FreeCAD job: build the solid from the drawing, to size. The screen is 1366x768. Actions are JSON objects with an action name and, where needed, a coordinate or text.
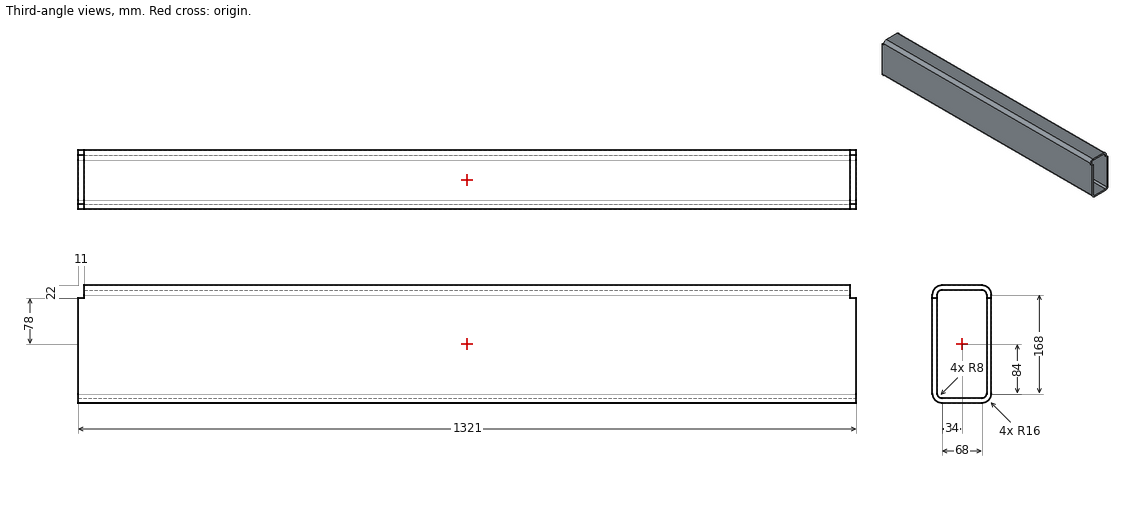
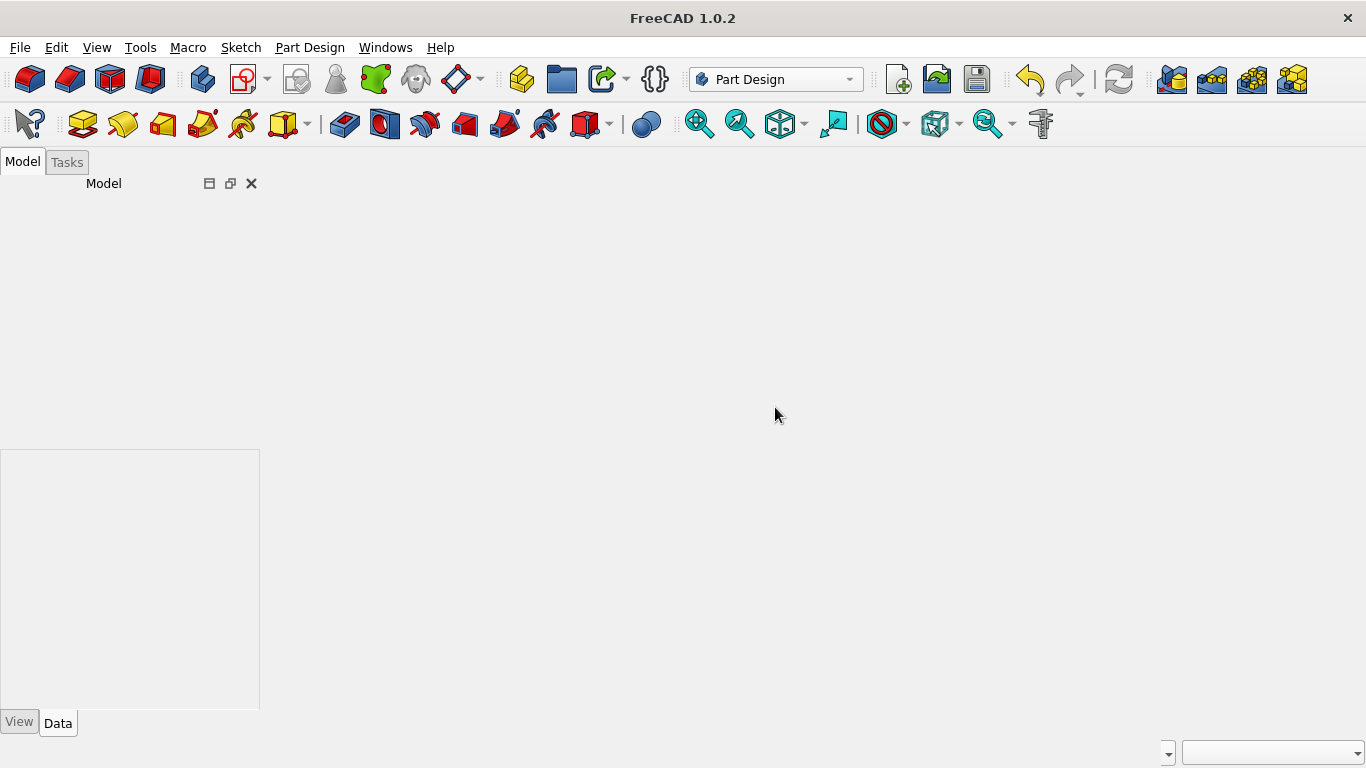
{"action": "left_click", "coordinate": [898, 80]}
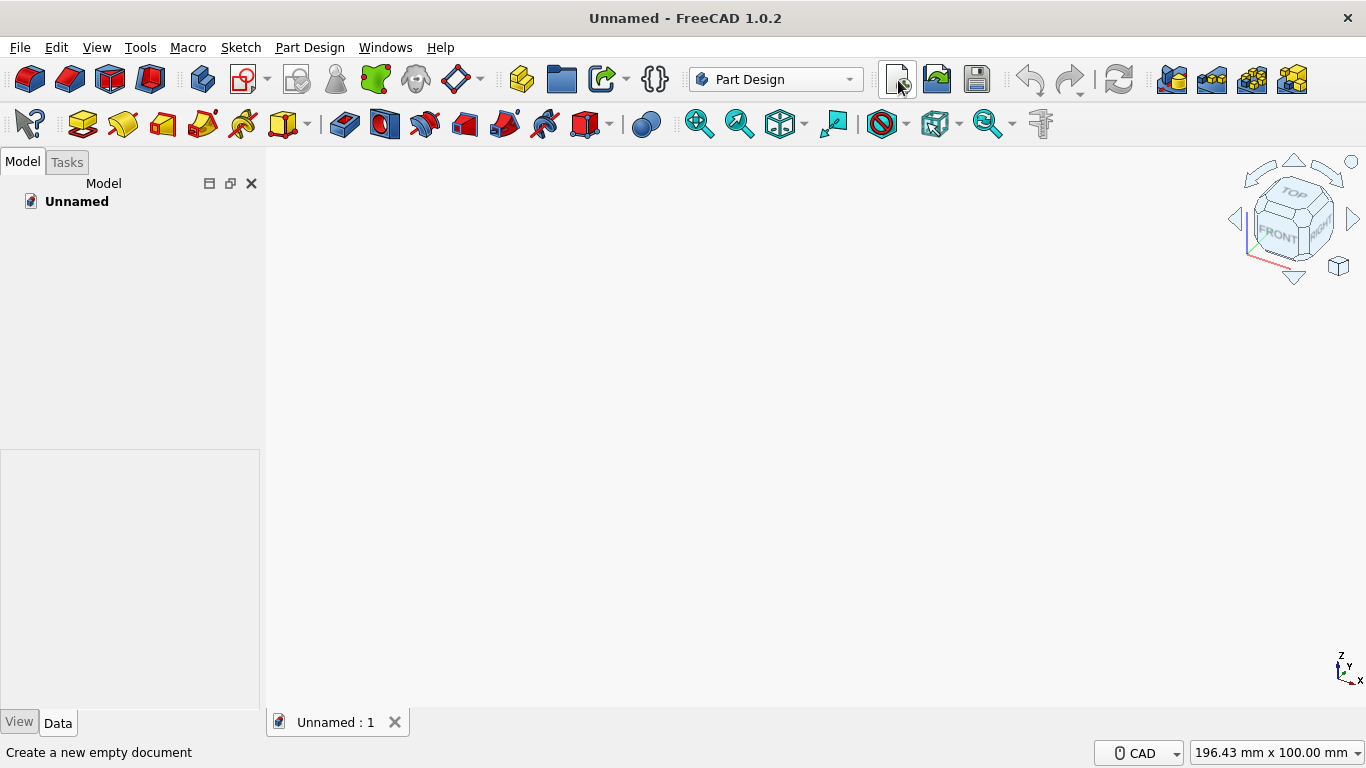
{"action": "left_click", "coordinate": [204, 80]}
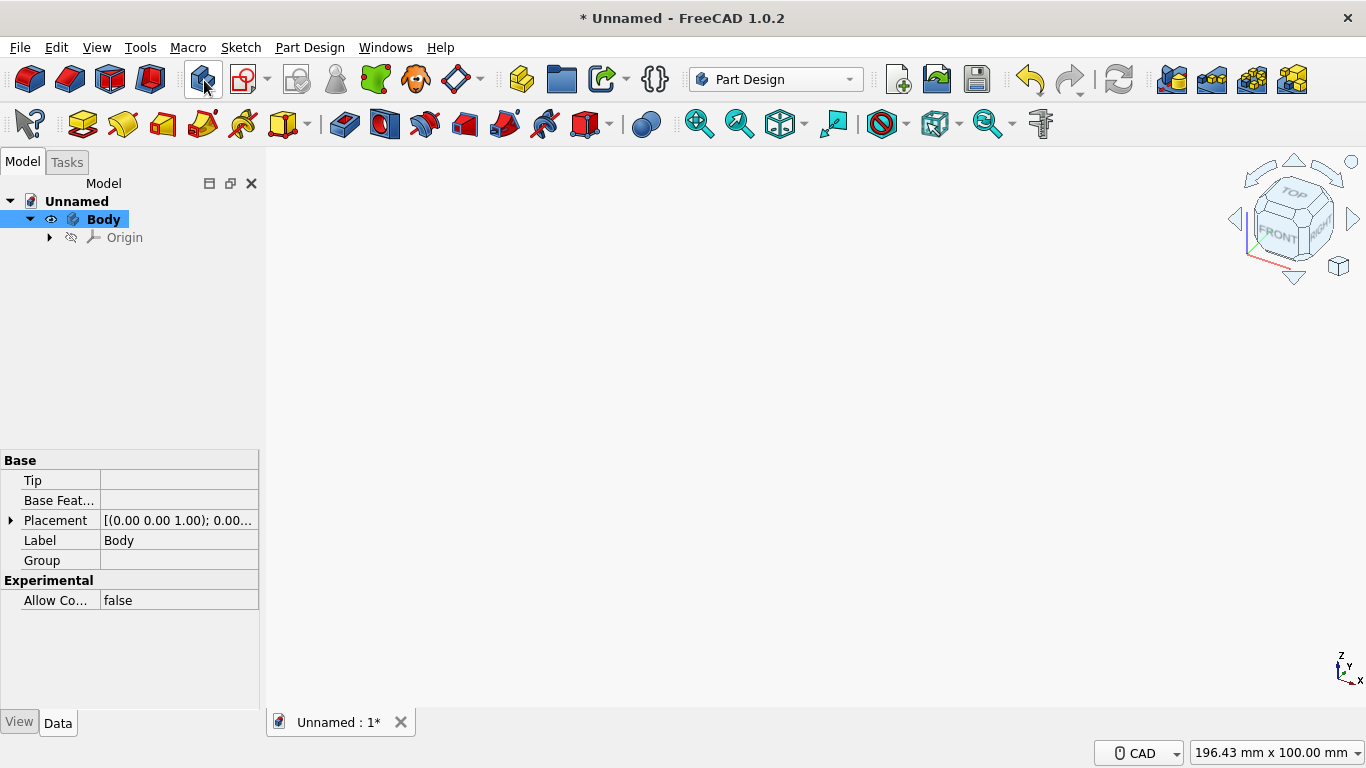
{"action": "left_click", "coordinate": [50, 237]}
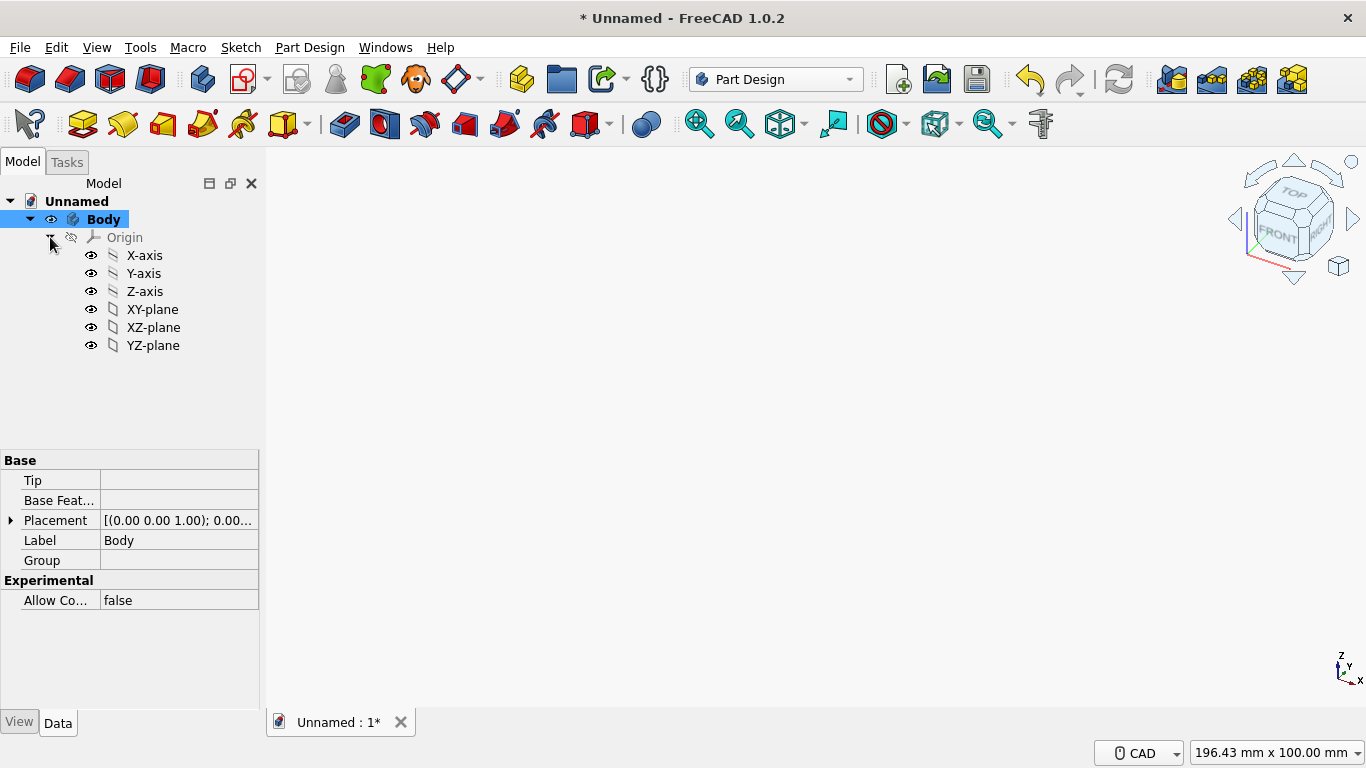
{"action": "left_click", "coordinate": [136, 345]}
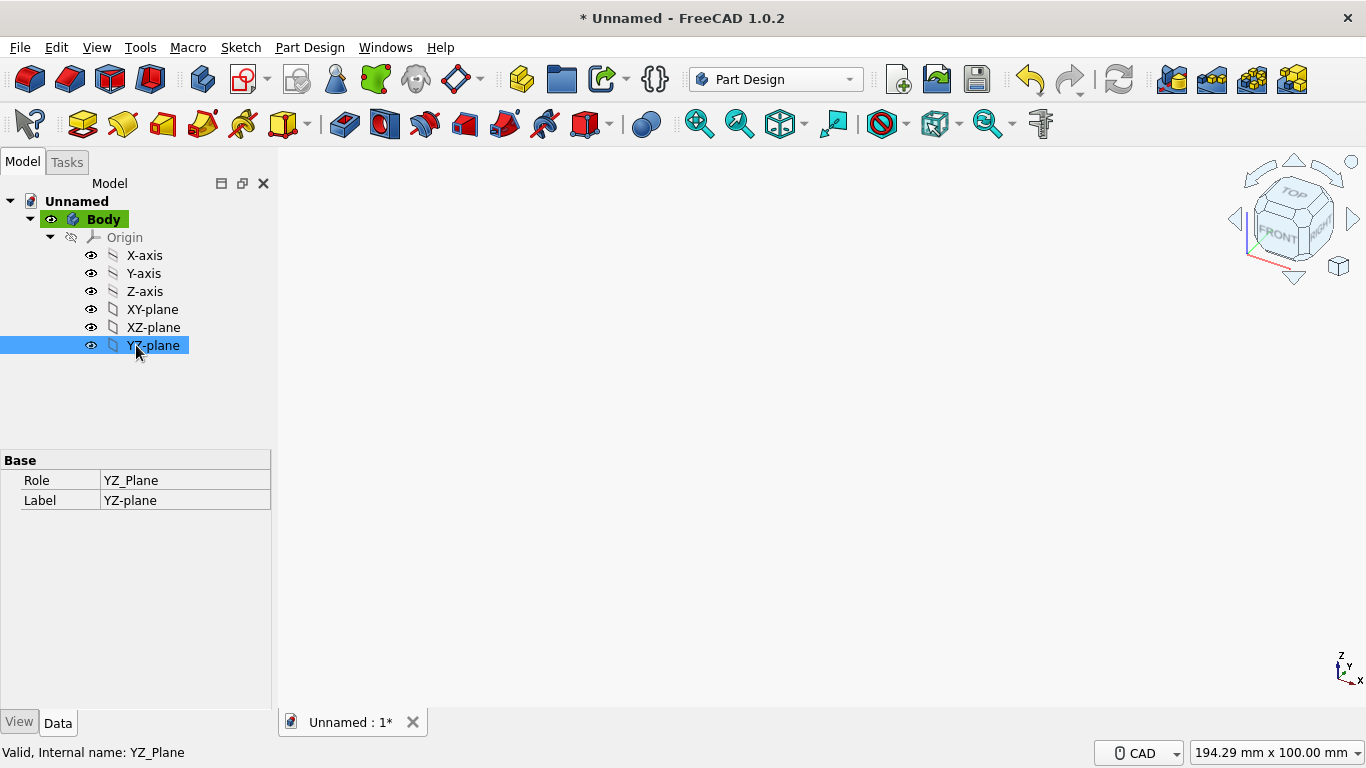
{"action": "left_click", "coordinate": [456, 80]}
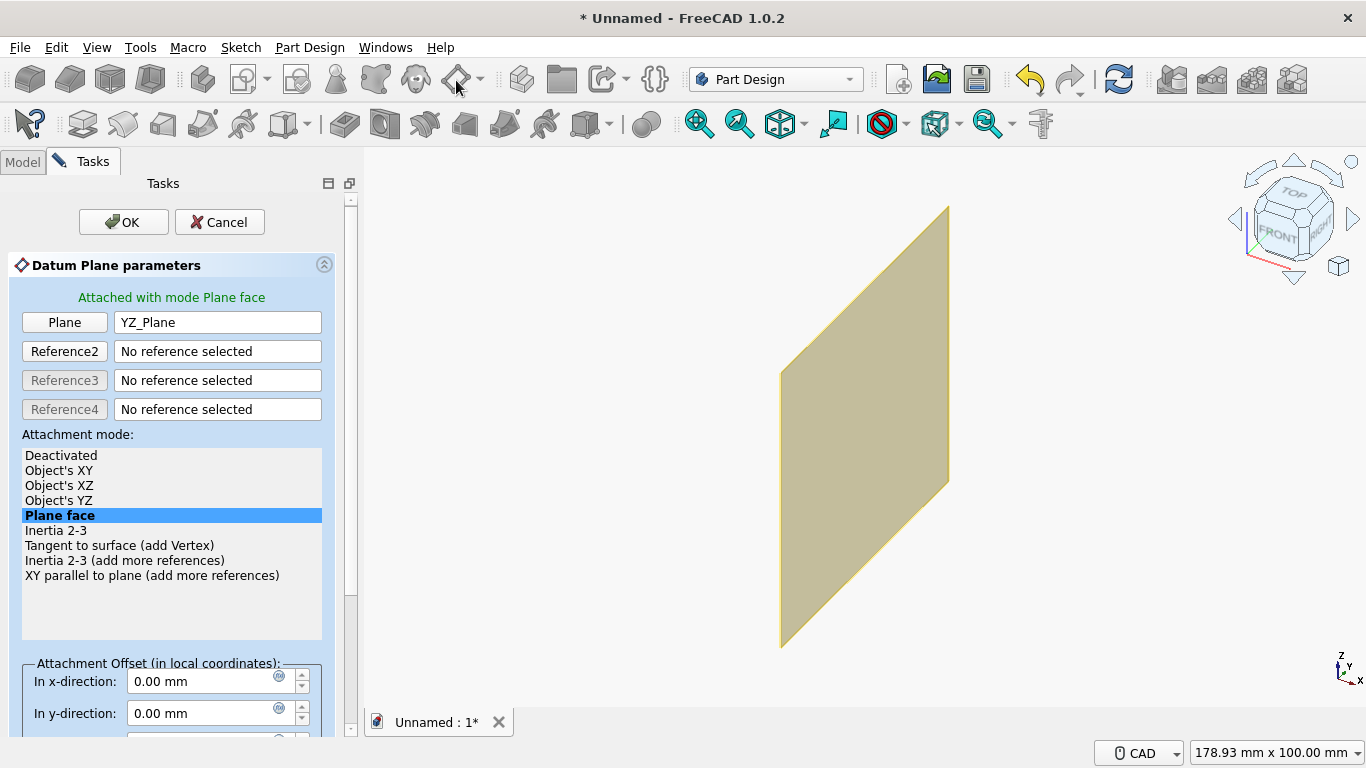
{"action": "scroll", "coordinate": [351, 464], "scroll_direction": "down", "scroll_amount": 2}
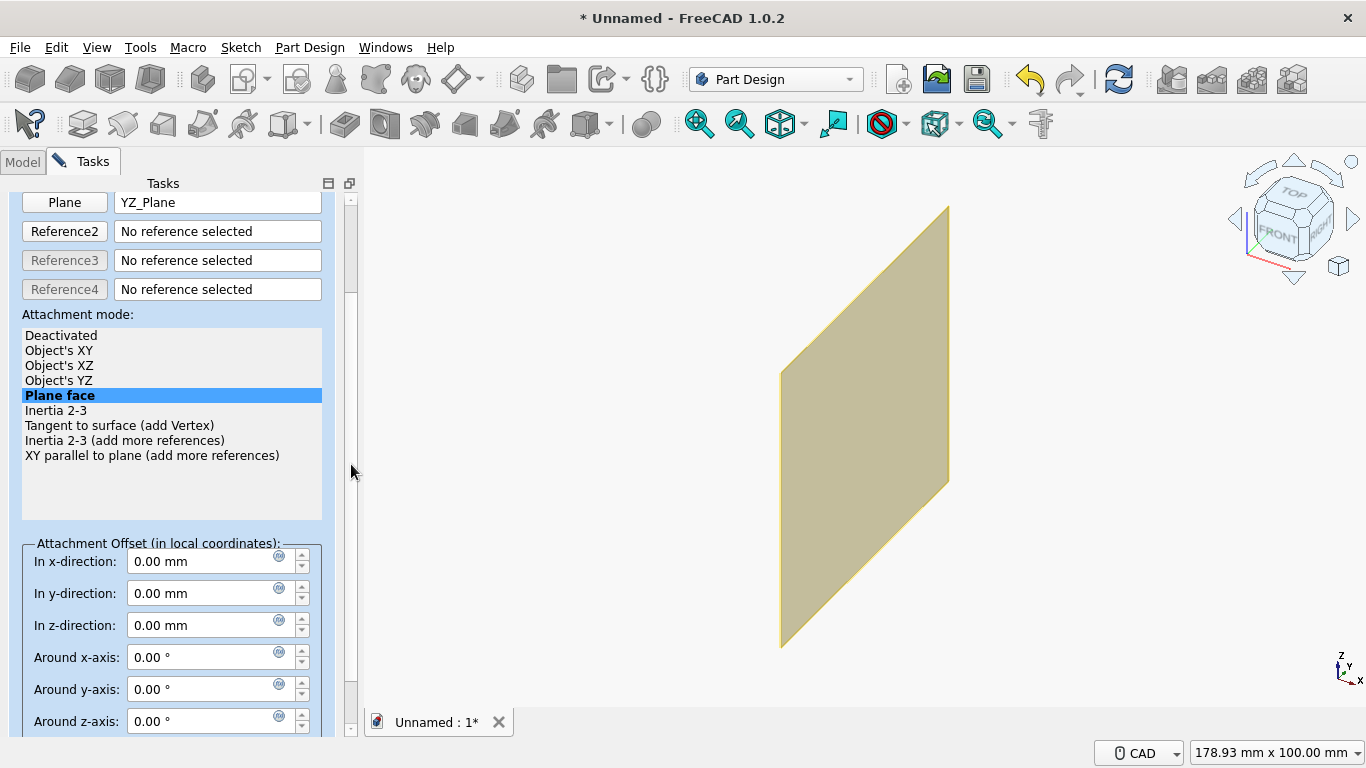
{"action": "triple_click", "coordinate": [210, 625]}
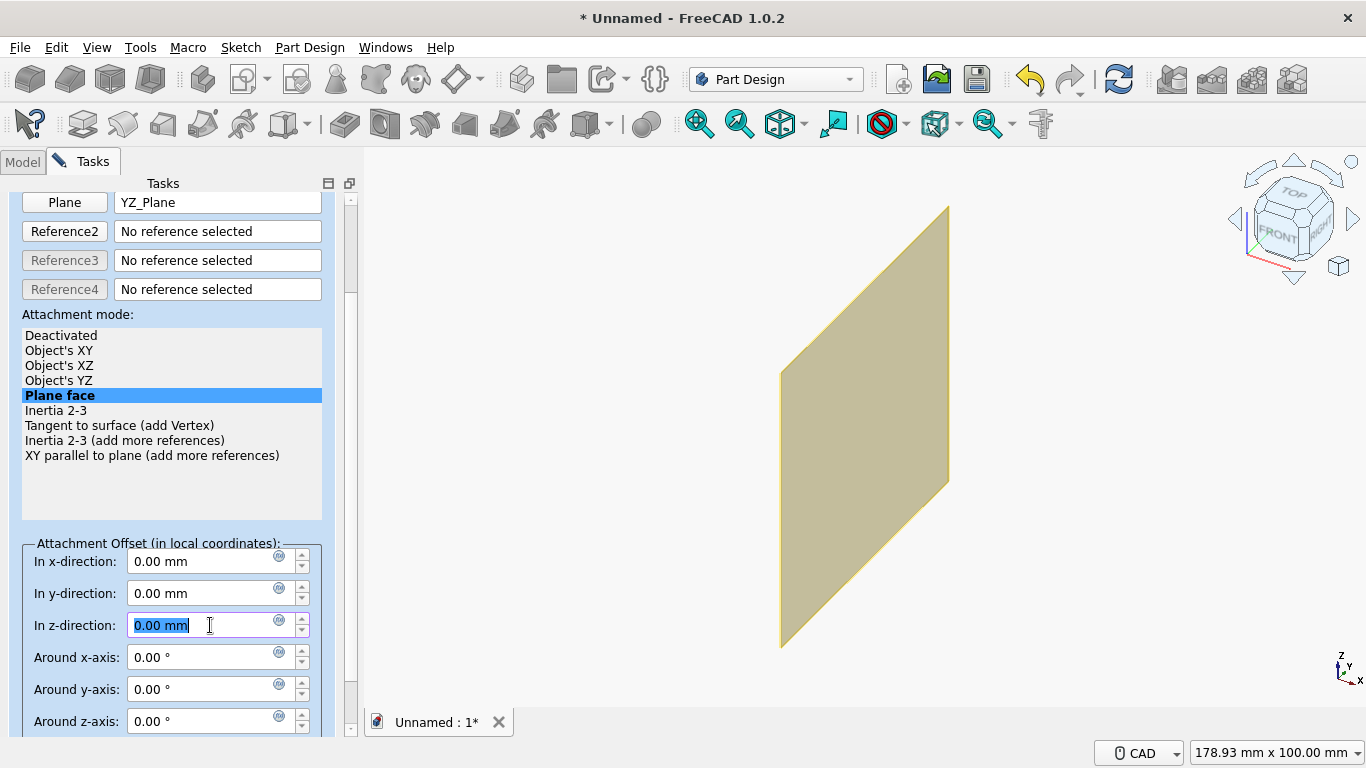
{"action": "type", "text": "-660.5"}
{"action": "key", "text": "Tab"}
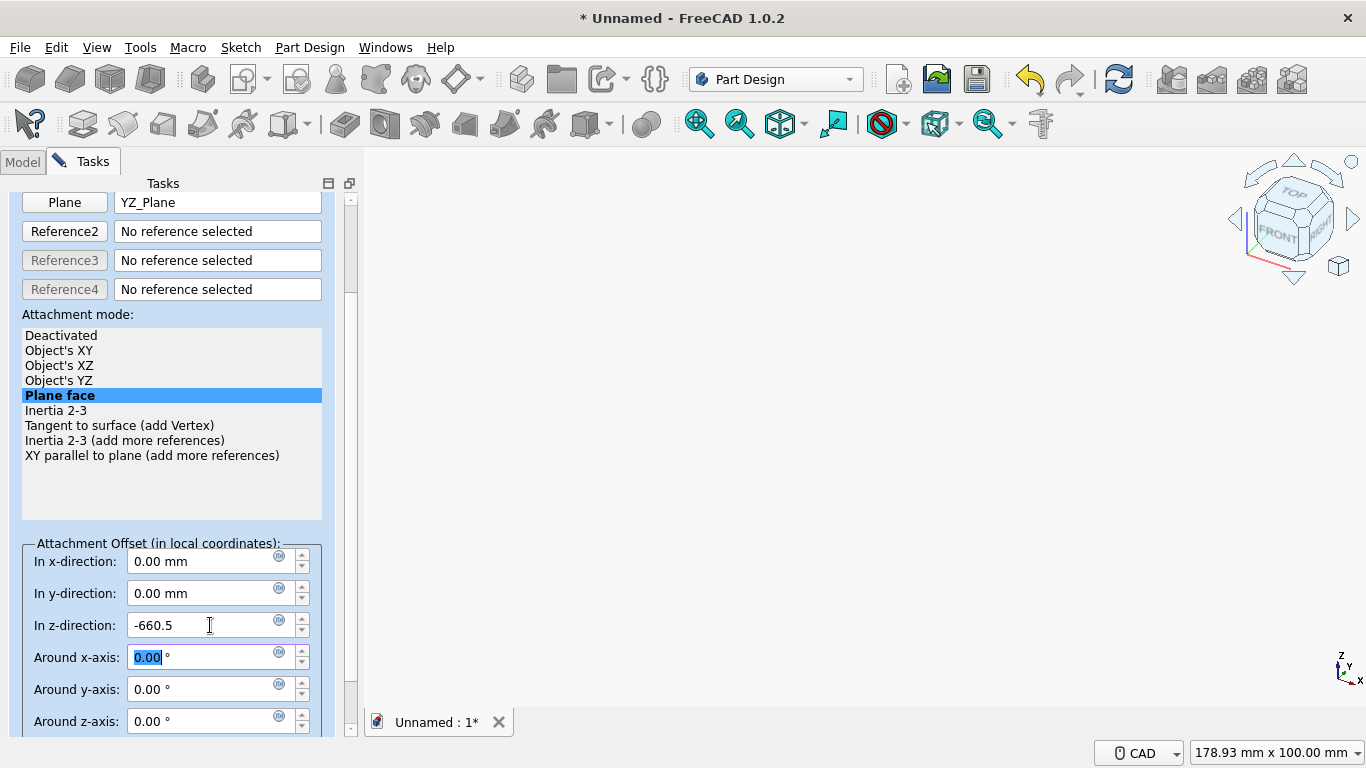
{"action": "scroll", "coordinate": [351, 464], "scroll_direction": "up", "scroll_amount": 3}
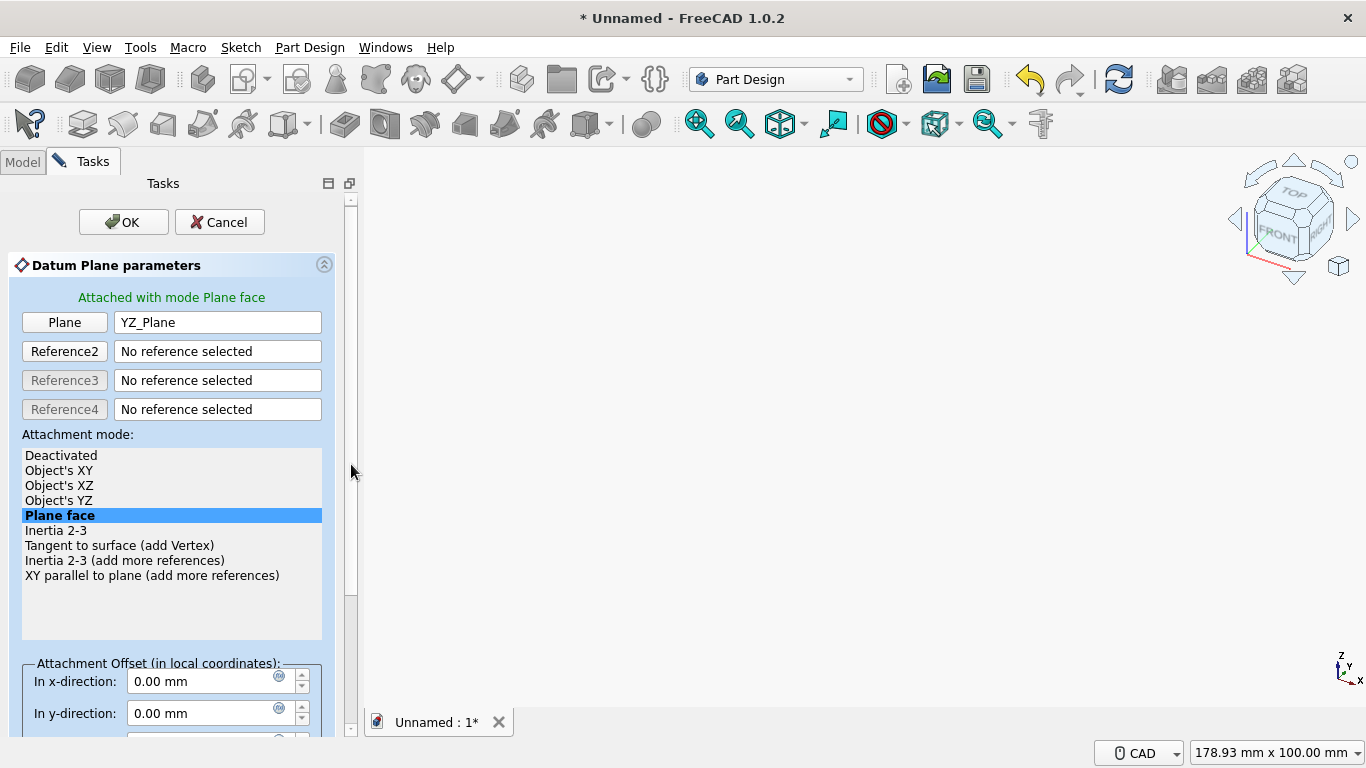
{"action": "left_click", "coordinate": [124, 222]}